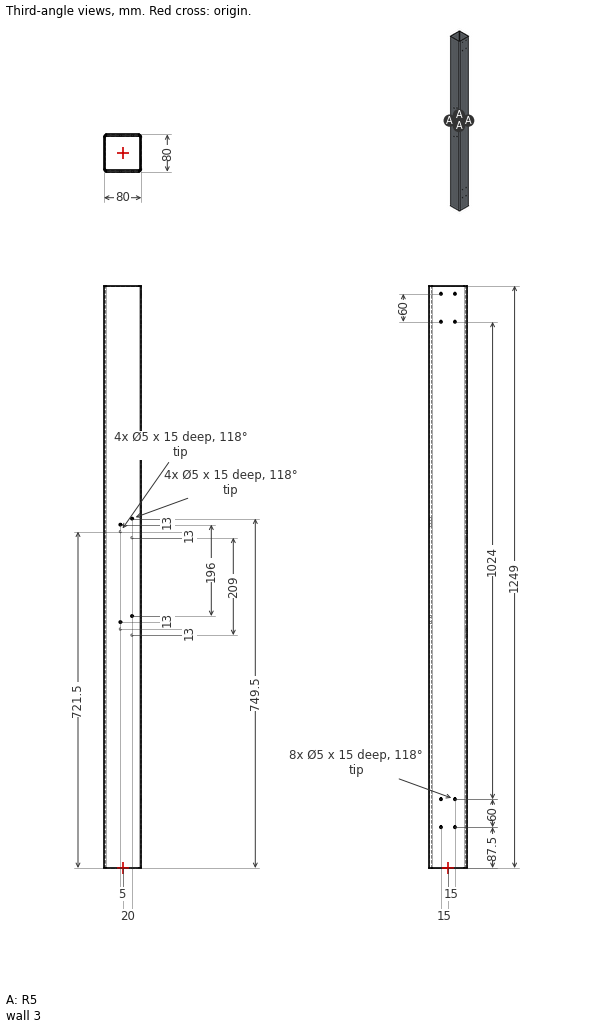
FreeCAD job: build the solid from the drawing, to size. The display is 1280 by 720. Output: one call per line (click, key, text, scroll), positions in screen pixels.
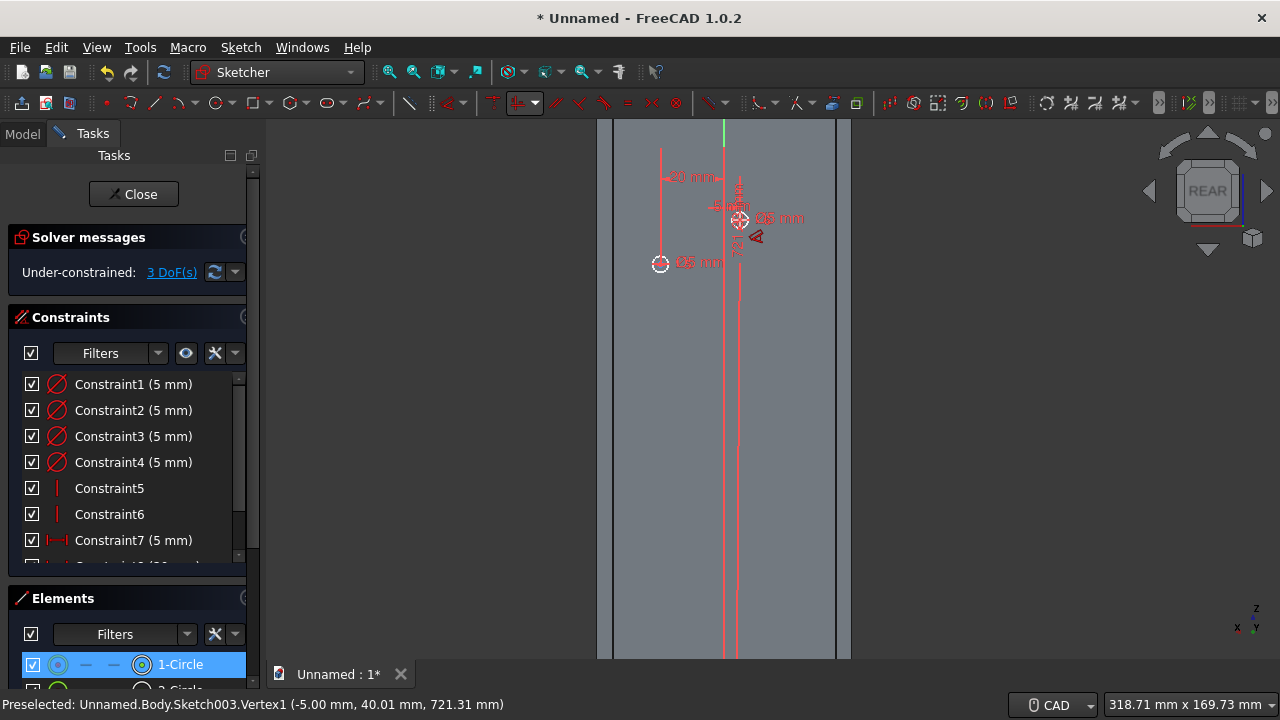
click(661, 264)
click(774, 242)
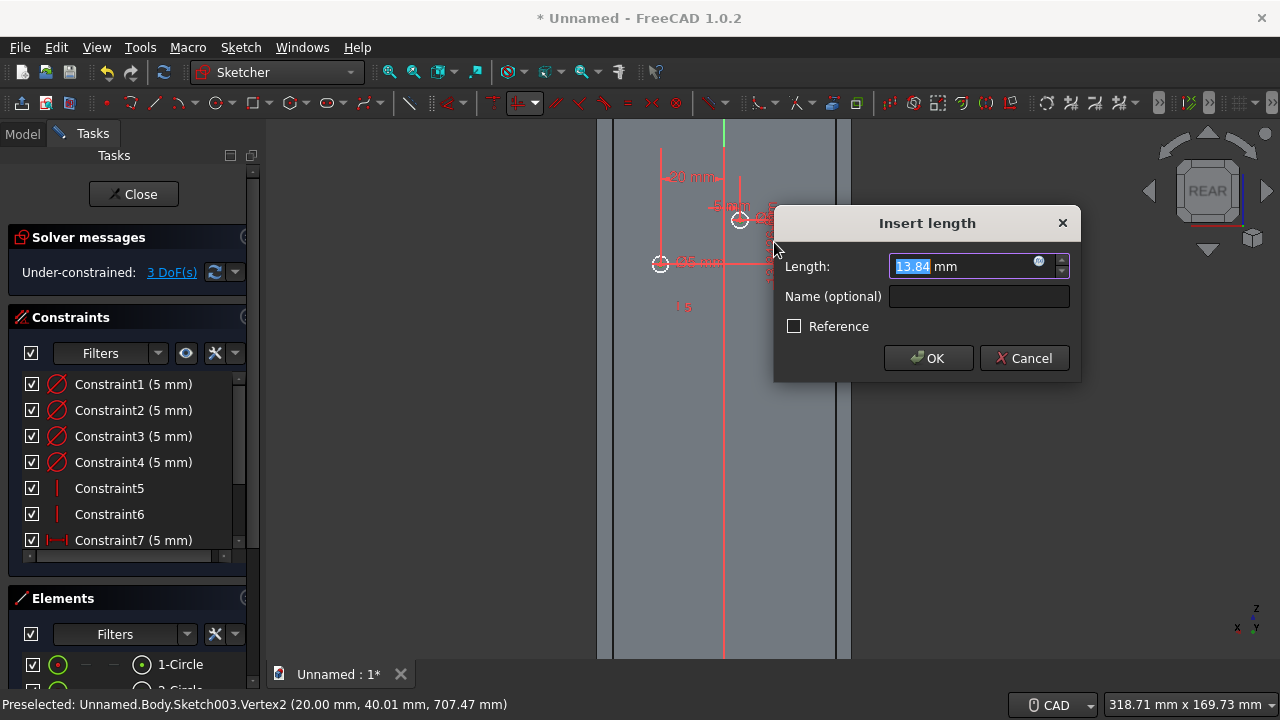
text(13)
key(Return)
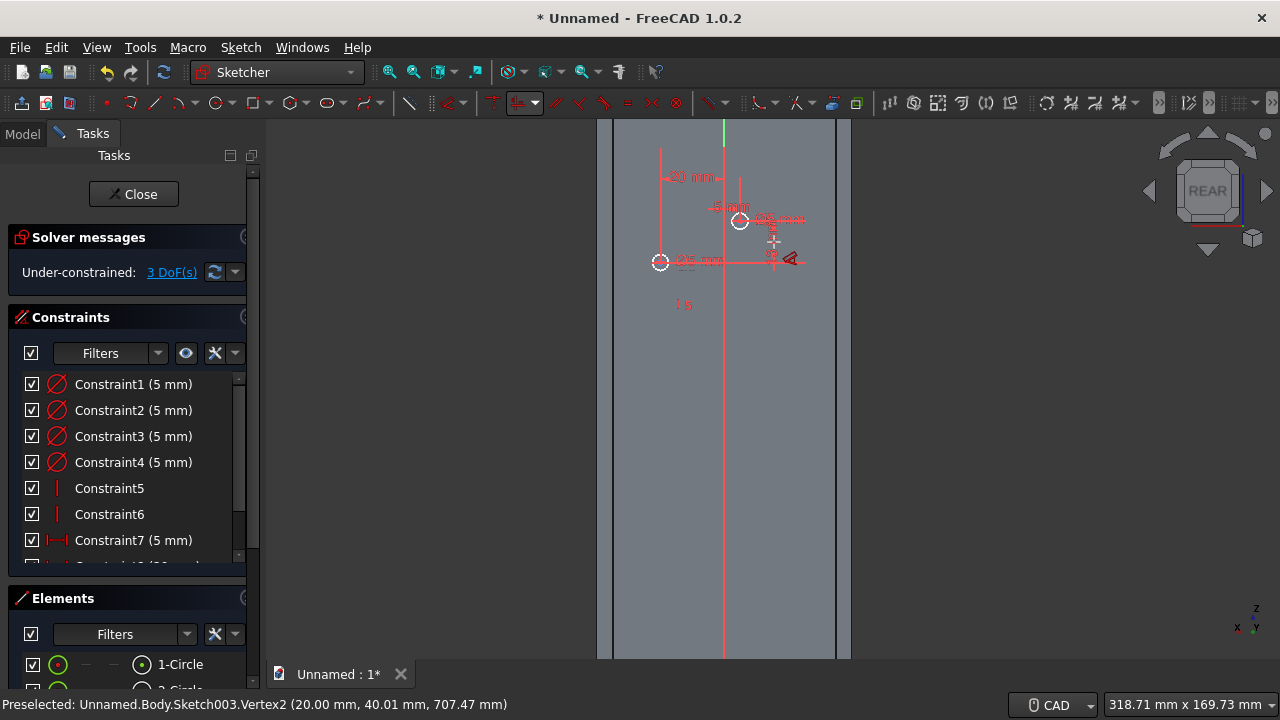
scroll(708, 239, down, 4)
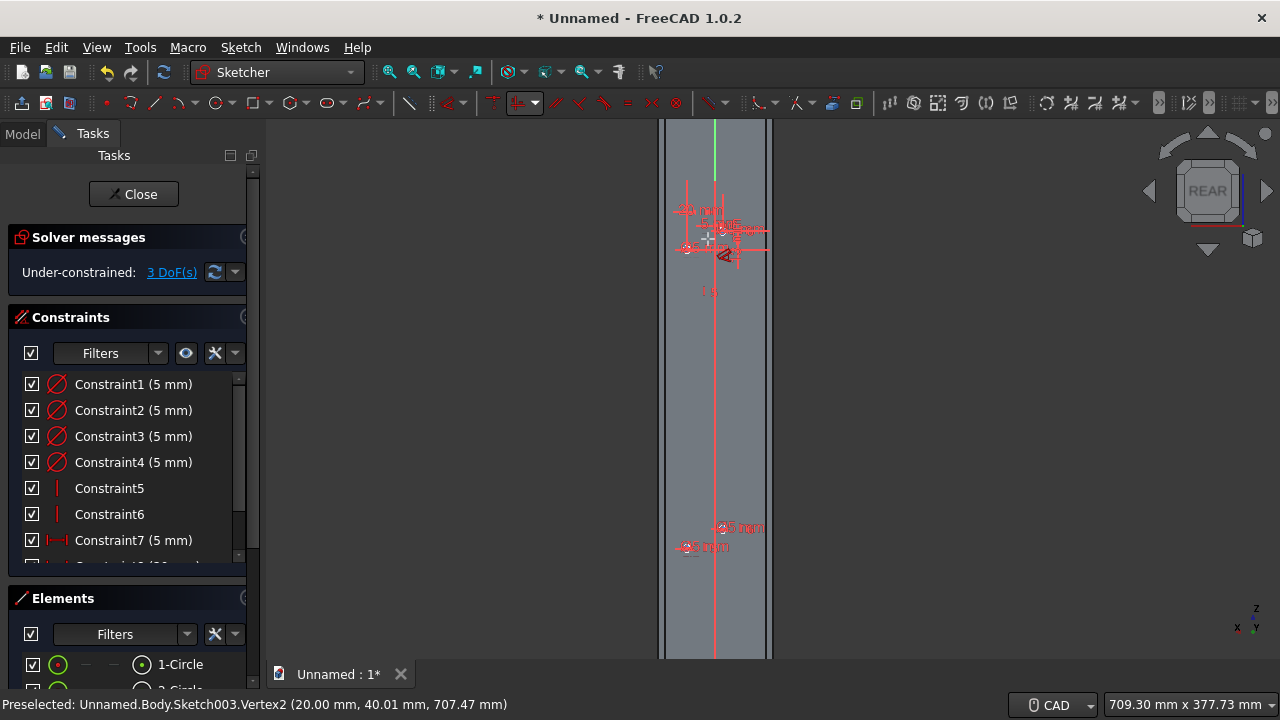
scroll(687, 549, up, 4)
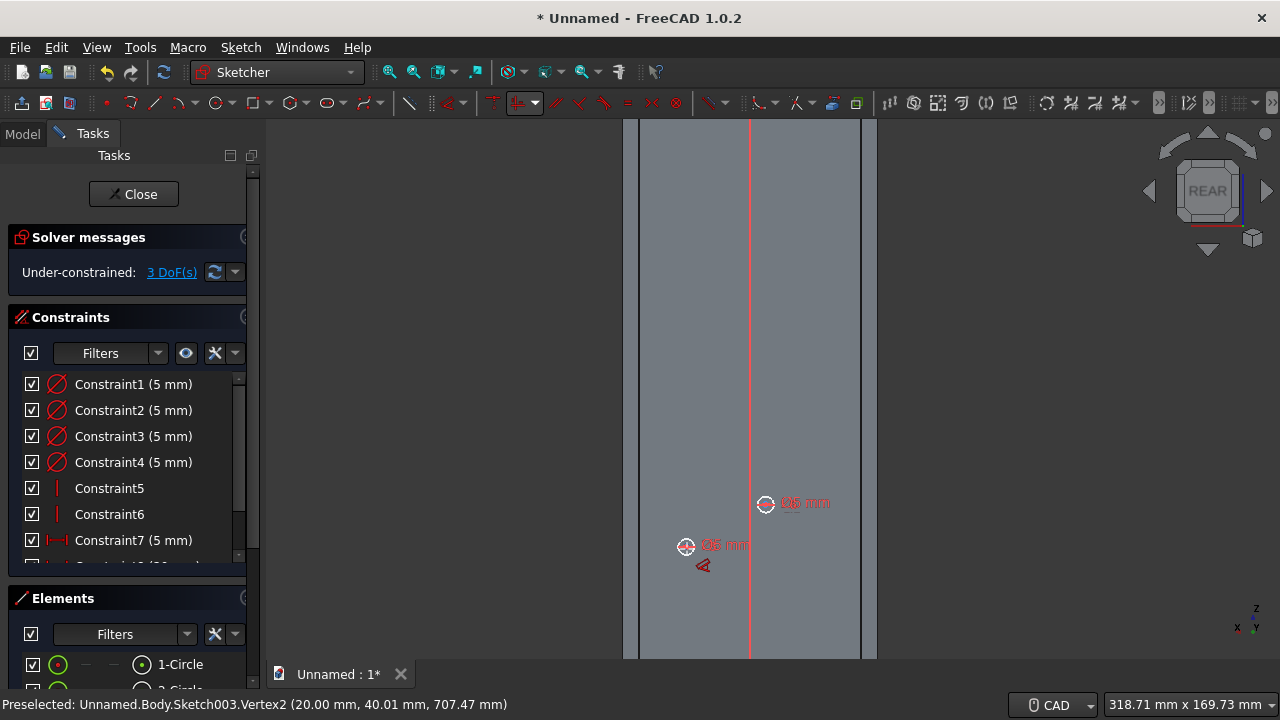
click(686, 547)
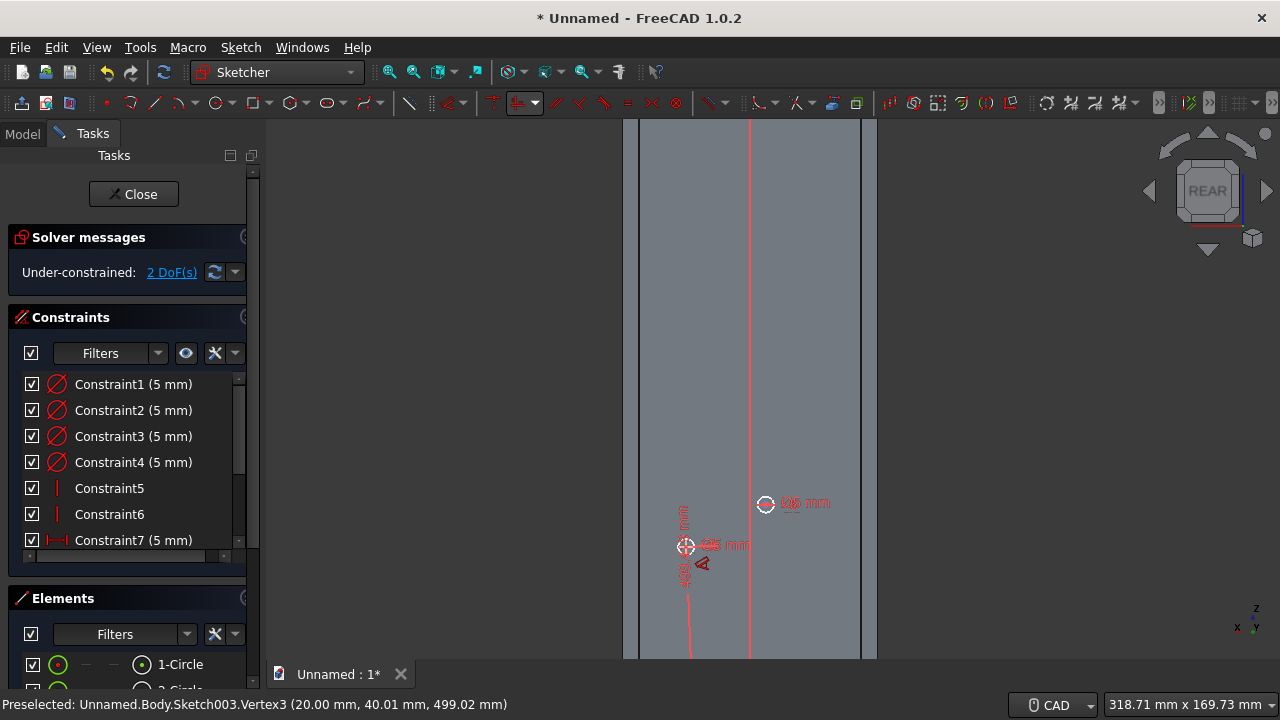
click(766, 505)
click(800, 526)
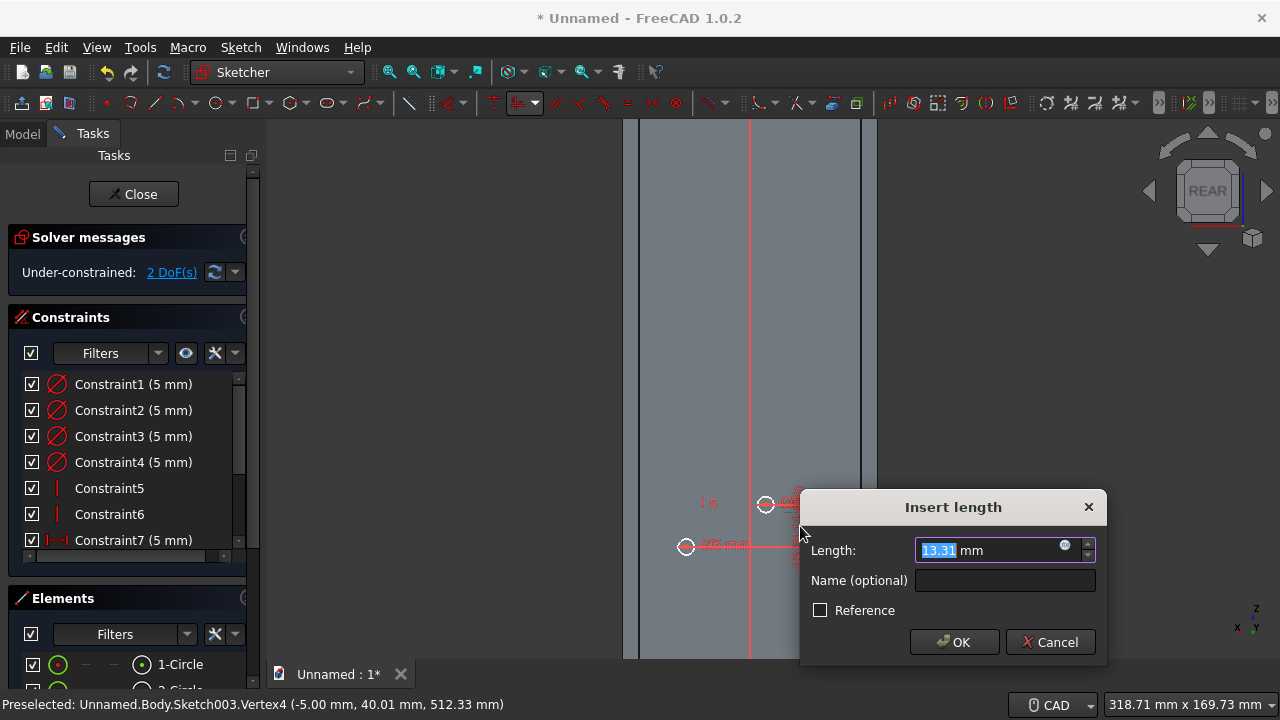
text(13)
key(Return)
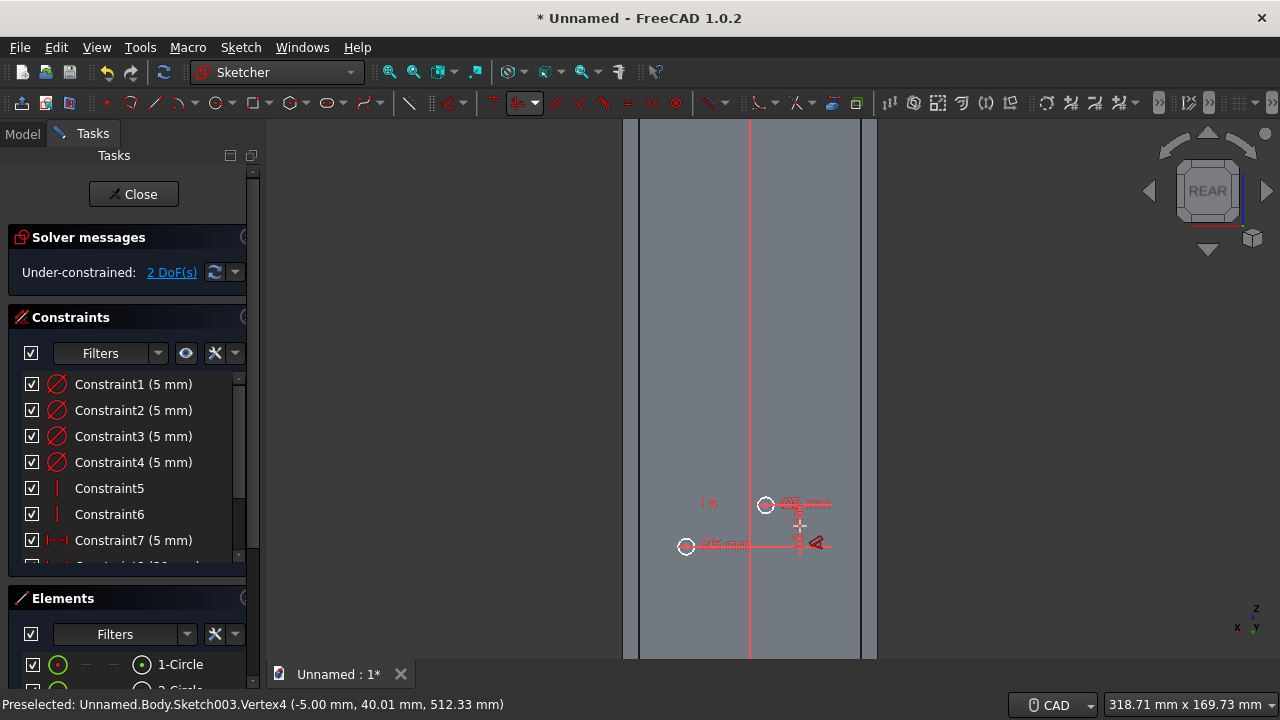
scroll(687, 550, down, 4)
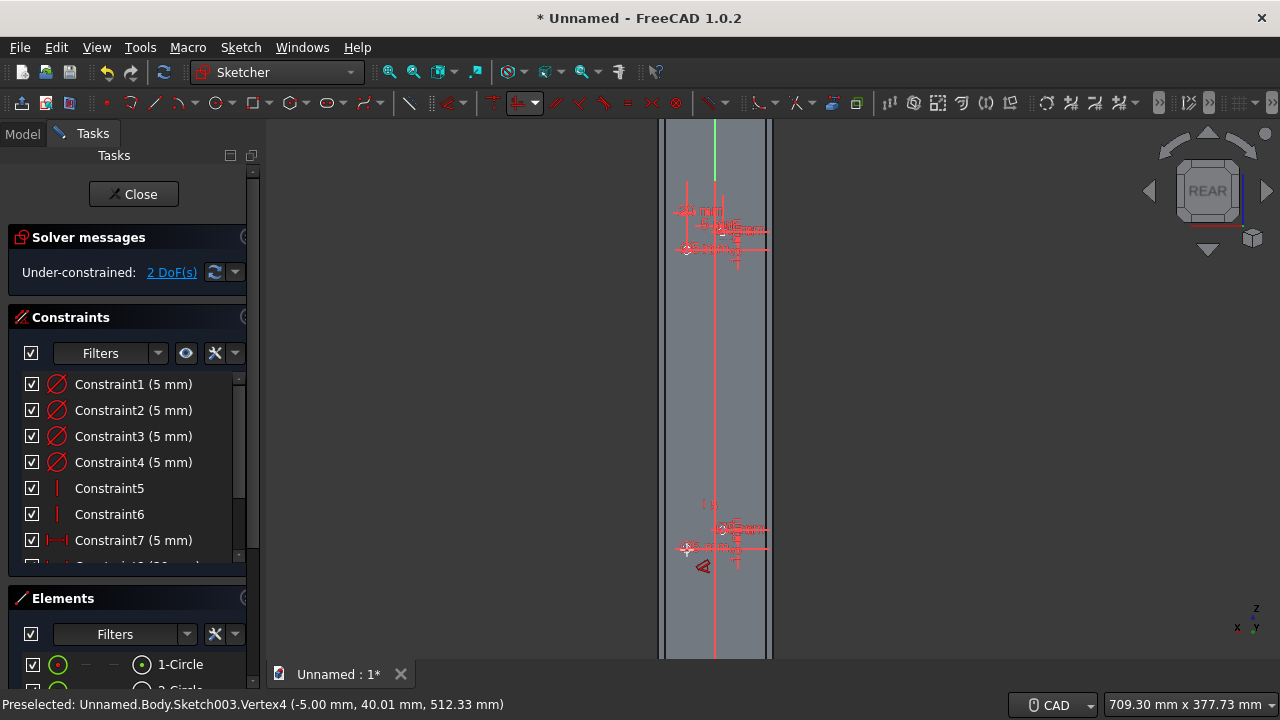
click(687, 250)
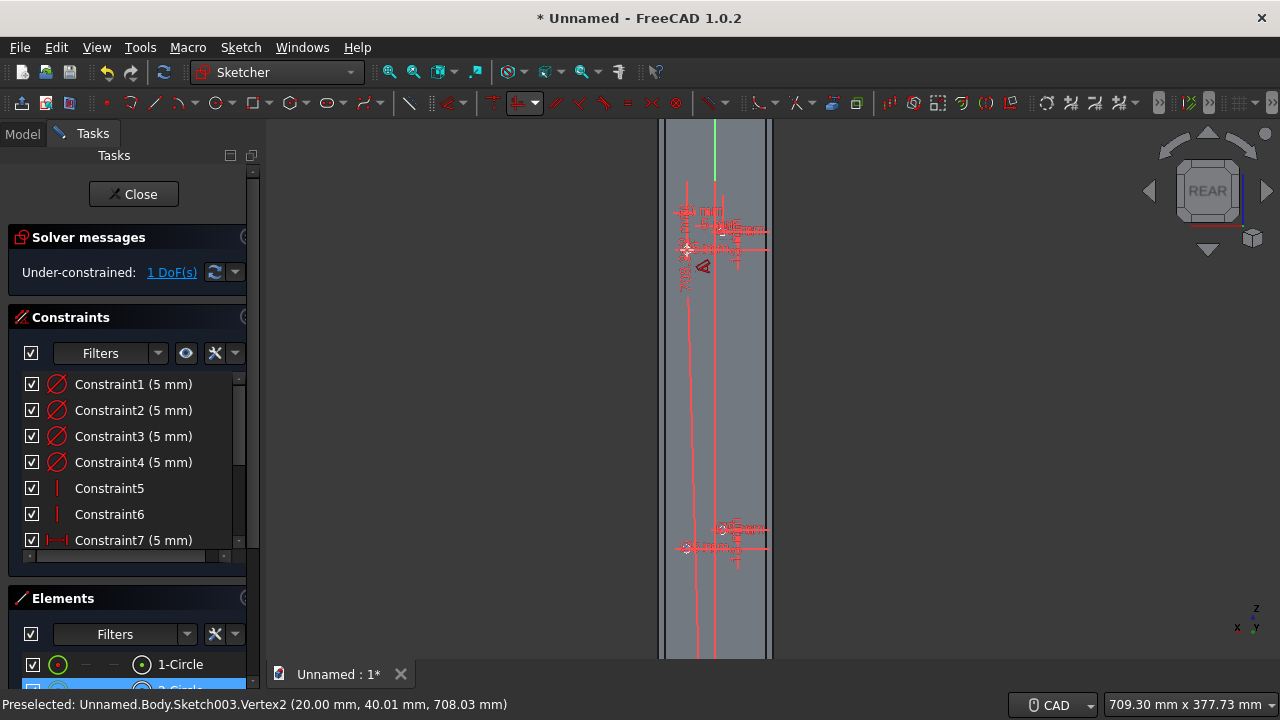
click(687, 549)
click(653, 400)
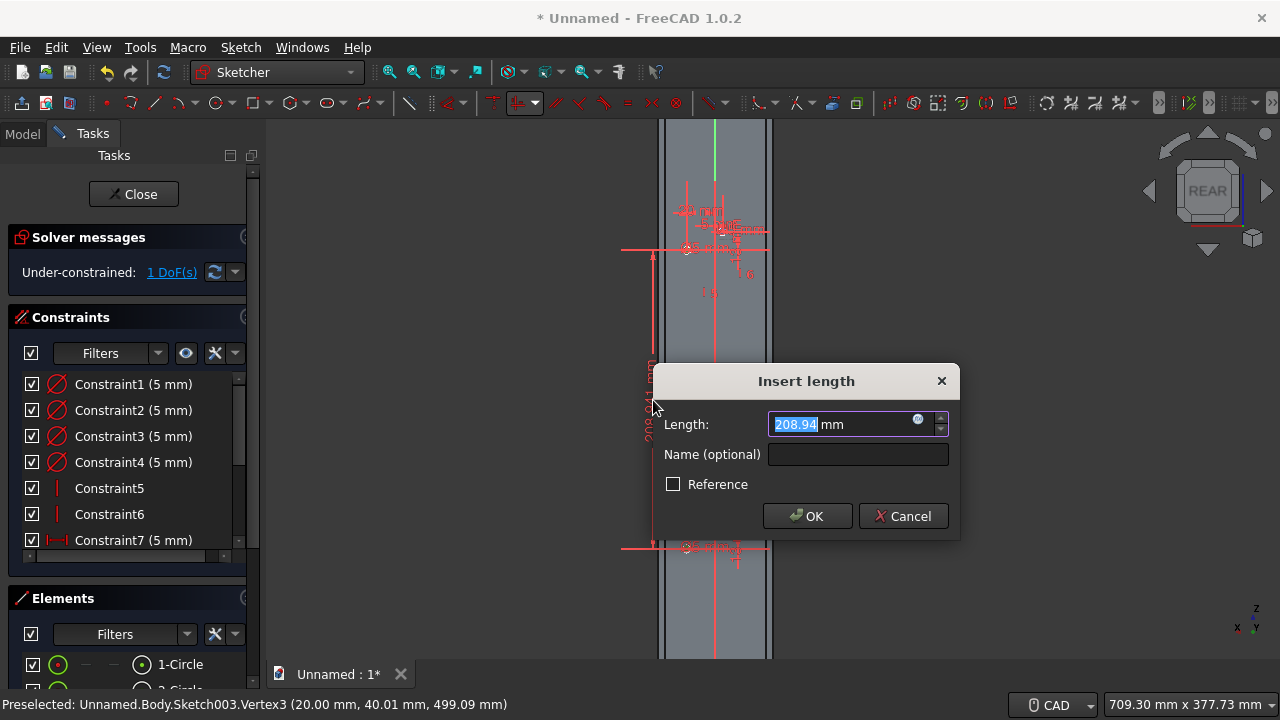
text(209)
key(Return)